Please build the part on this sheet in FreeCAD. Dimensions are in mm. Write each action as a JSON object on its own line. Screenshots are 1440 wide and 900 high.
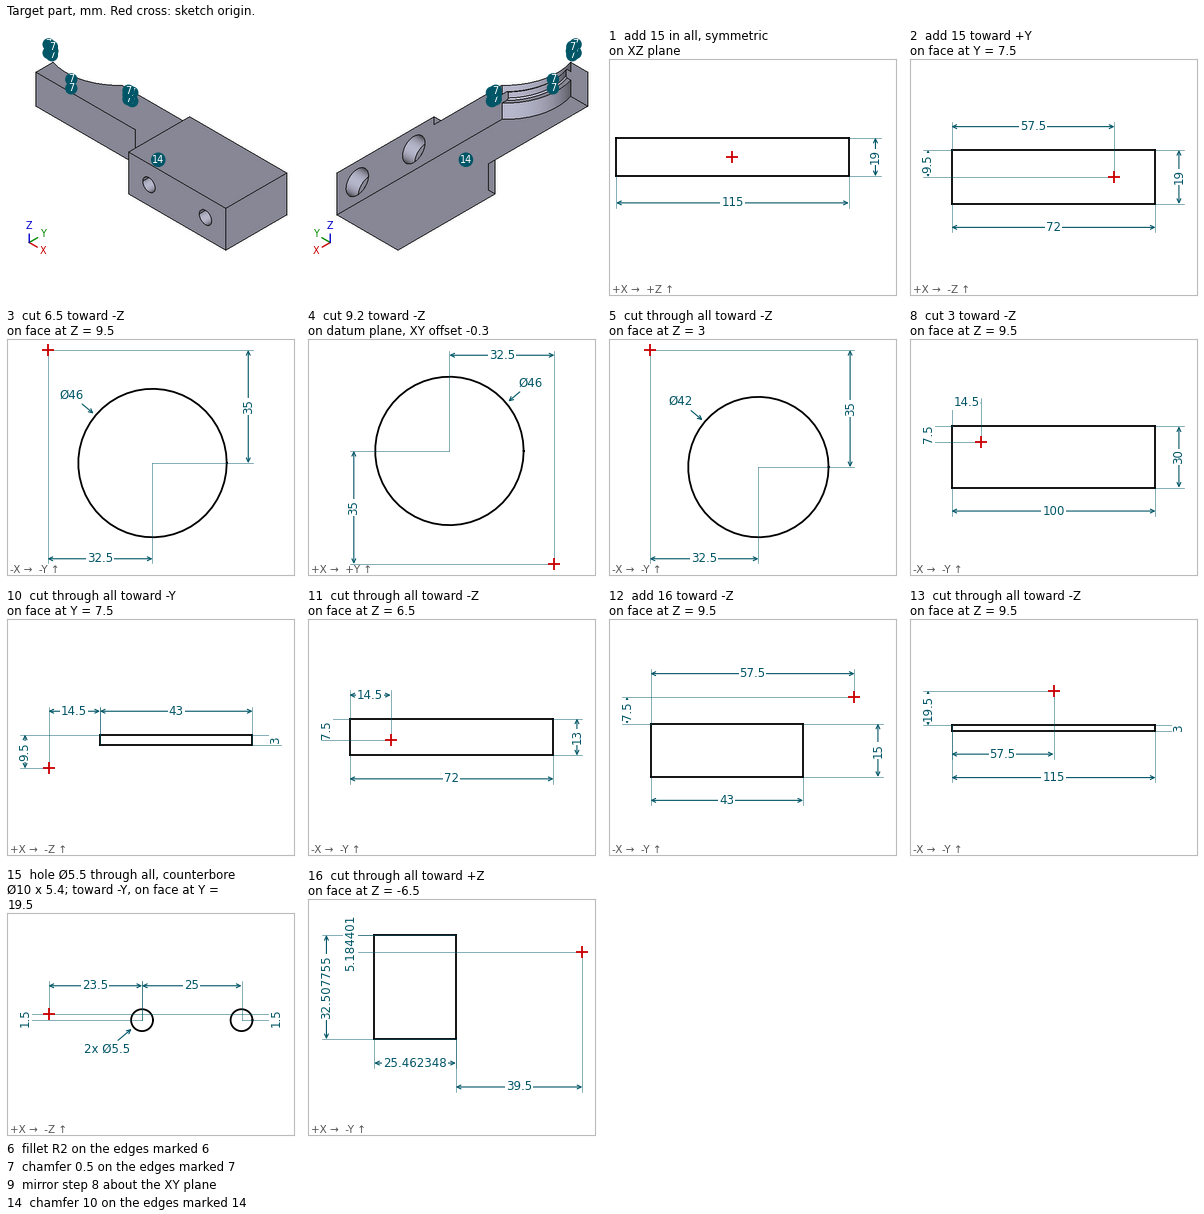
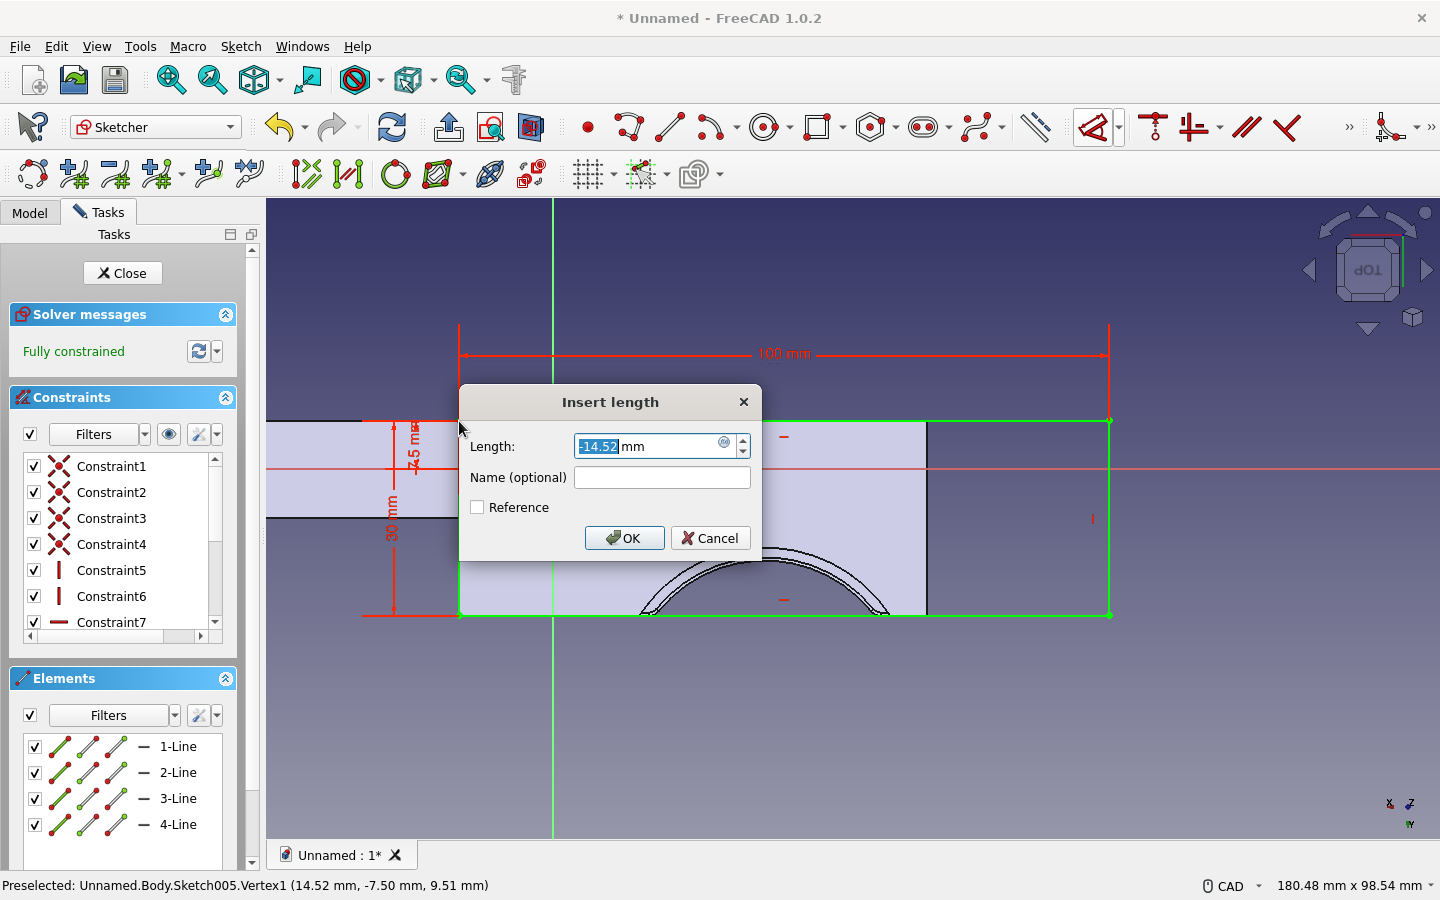
{"action": "type", "text": "-14.5"}
{"action": "key", "text": "Return"}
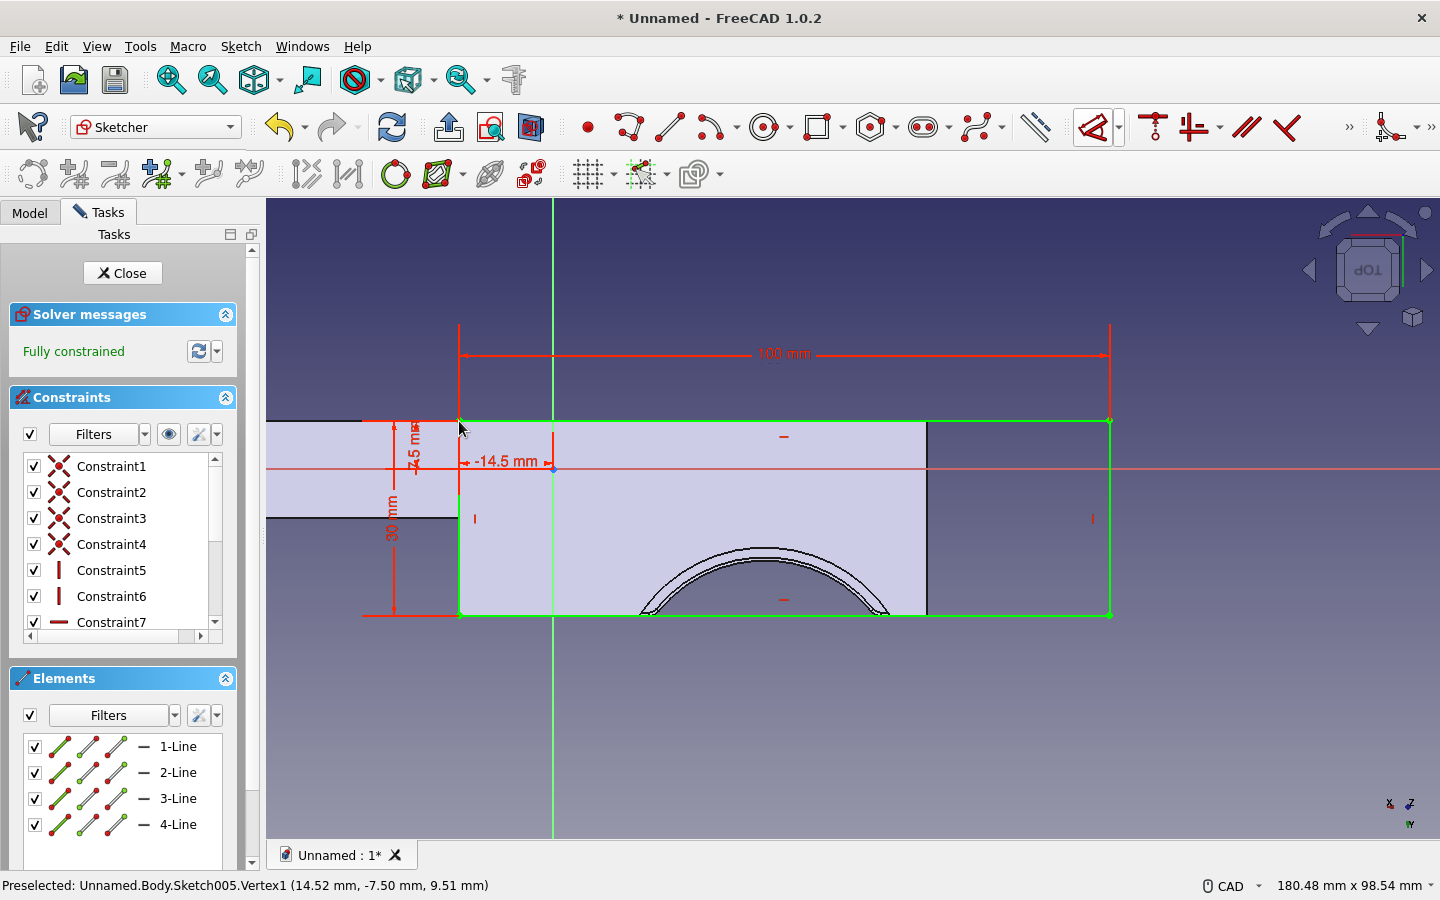
{"action": "left_click", "coordinate": [123, 273]}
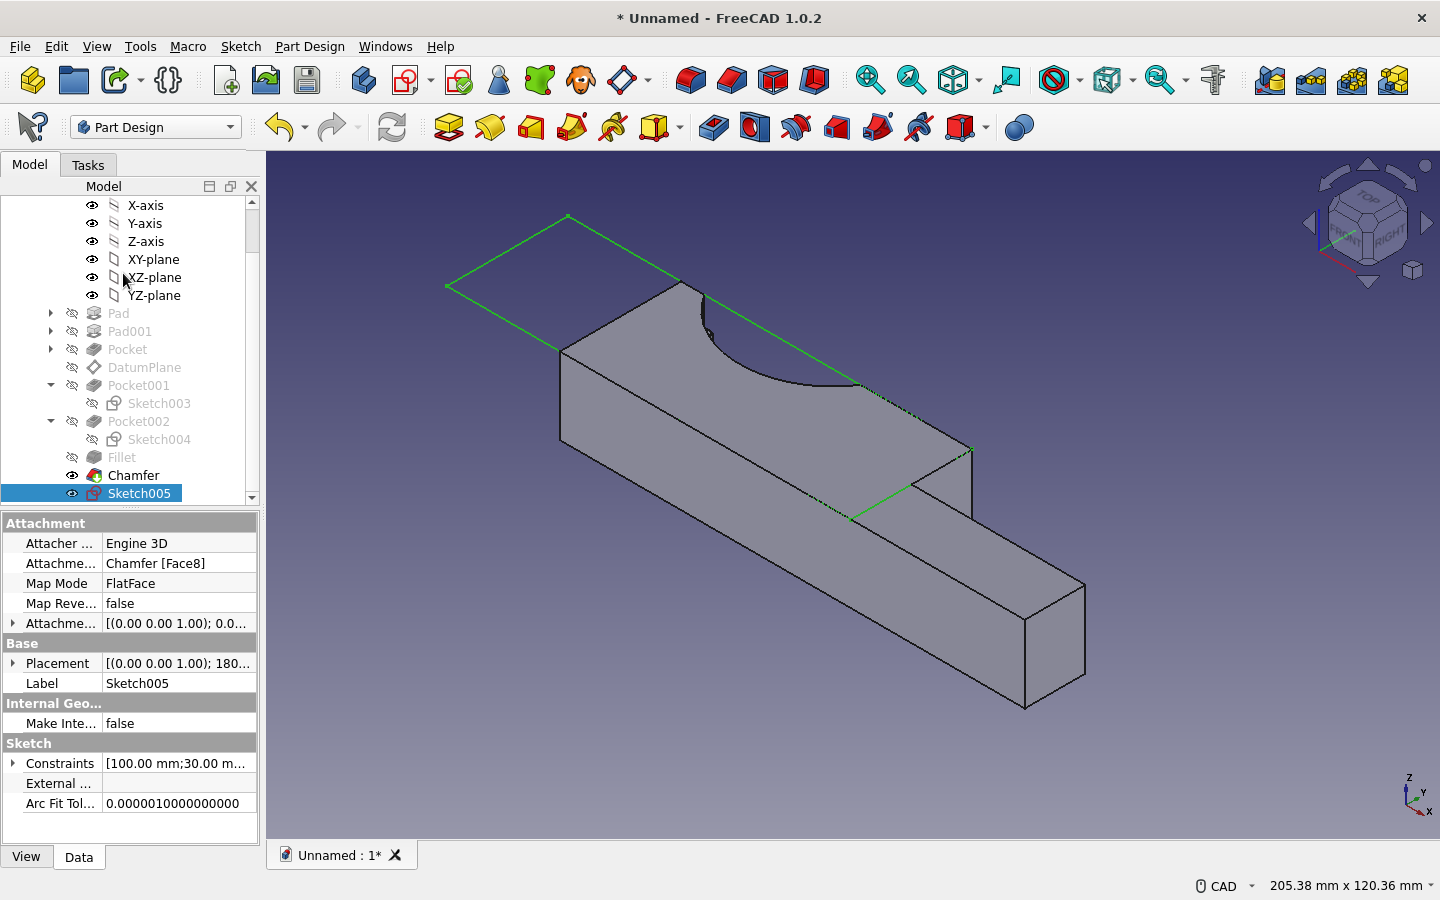
{"action": "left_click", "coordinate": [714, 128]}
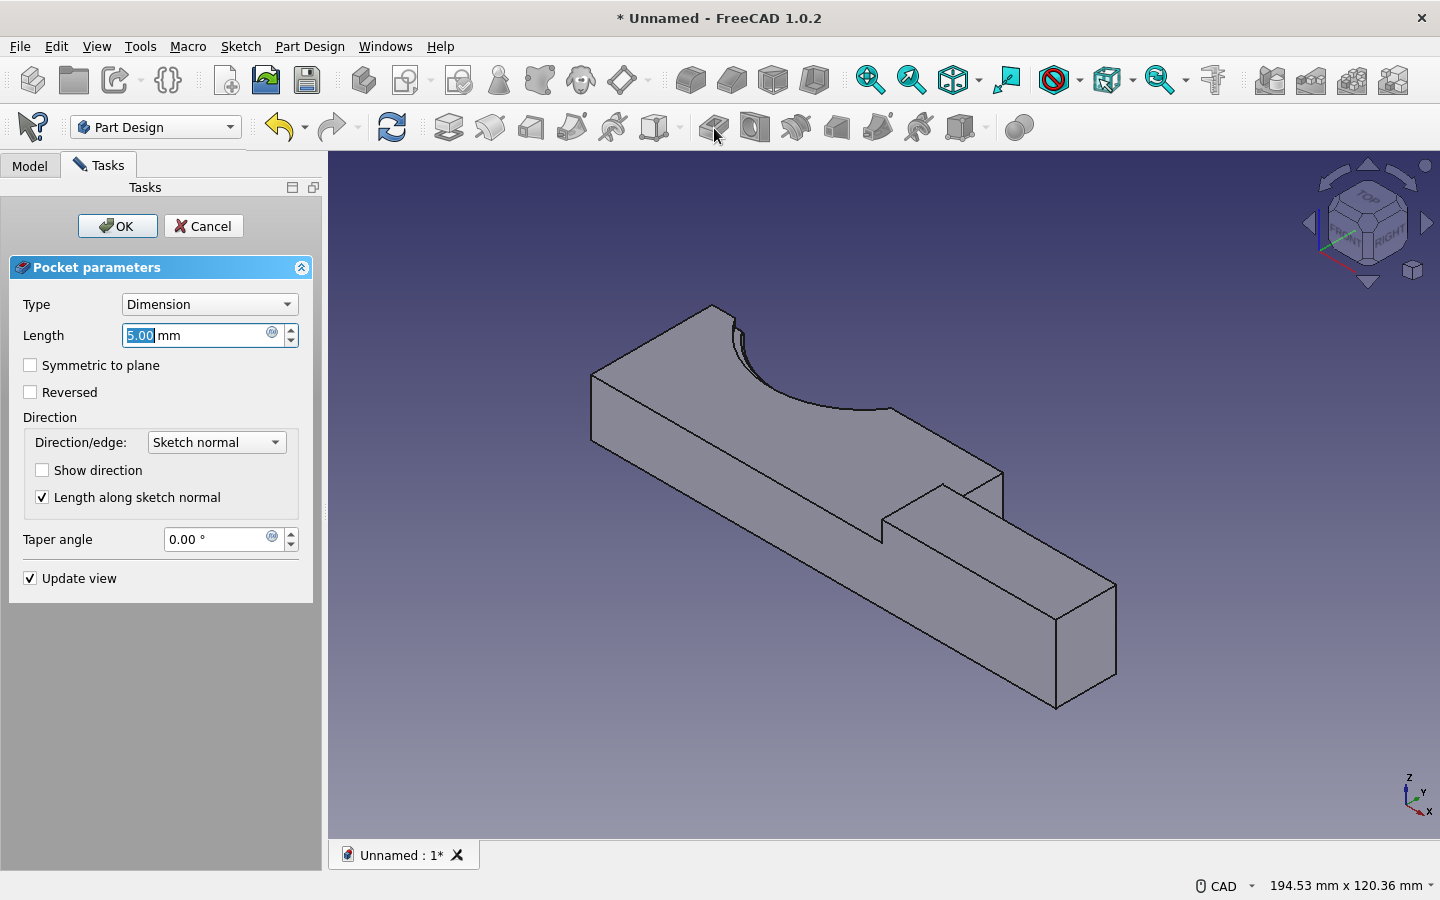
{"action": "type", "text": "3"}
{"action": "key", "text": "Tab"}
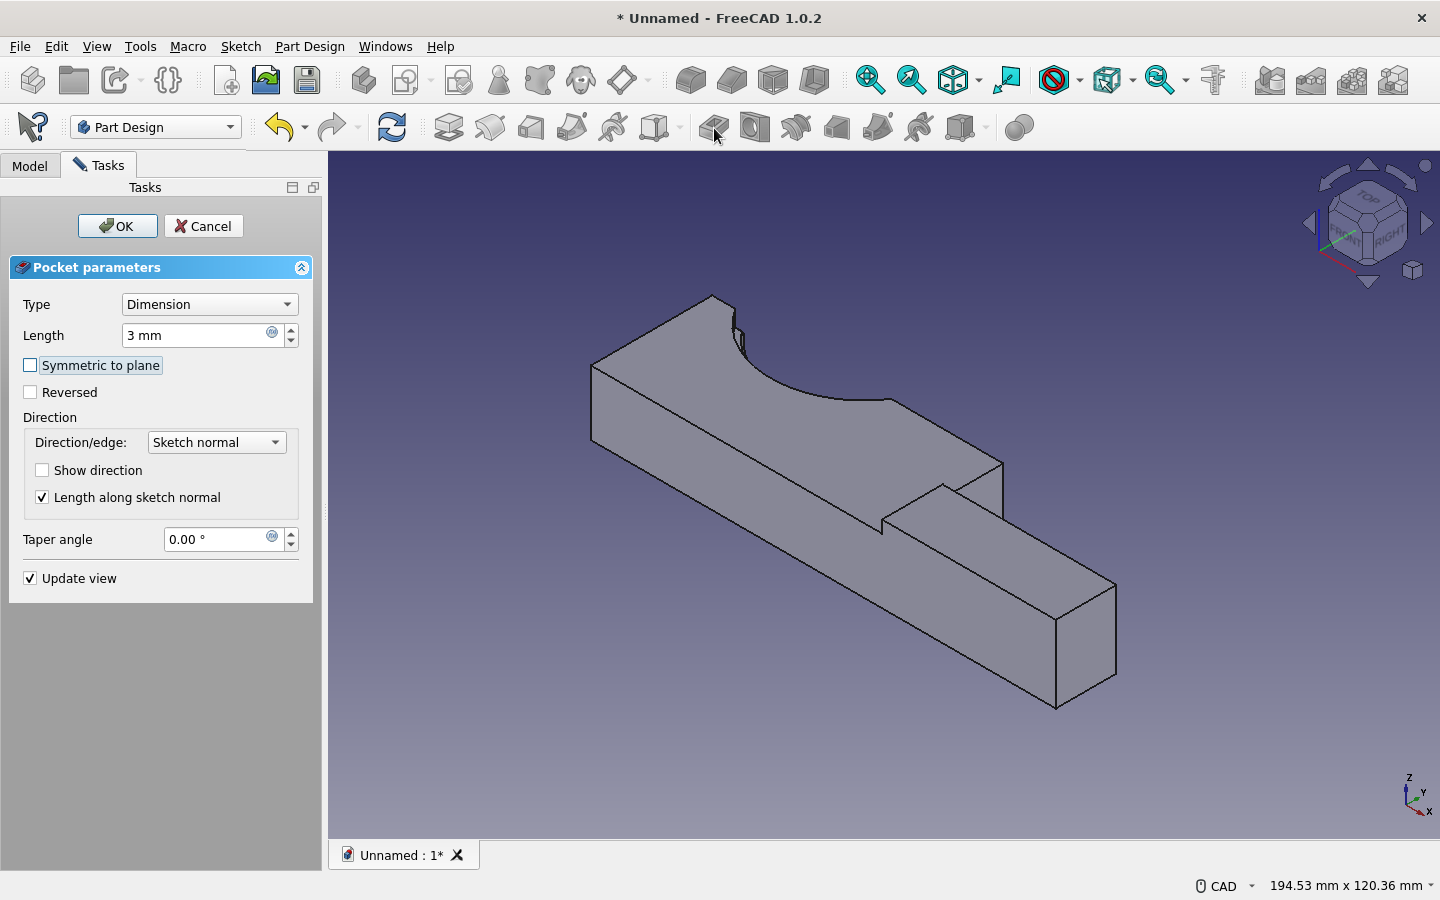
{"action": "left_click", "coordinate": [118, 226]}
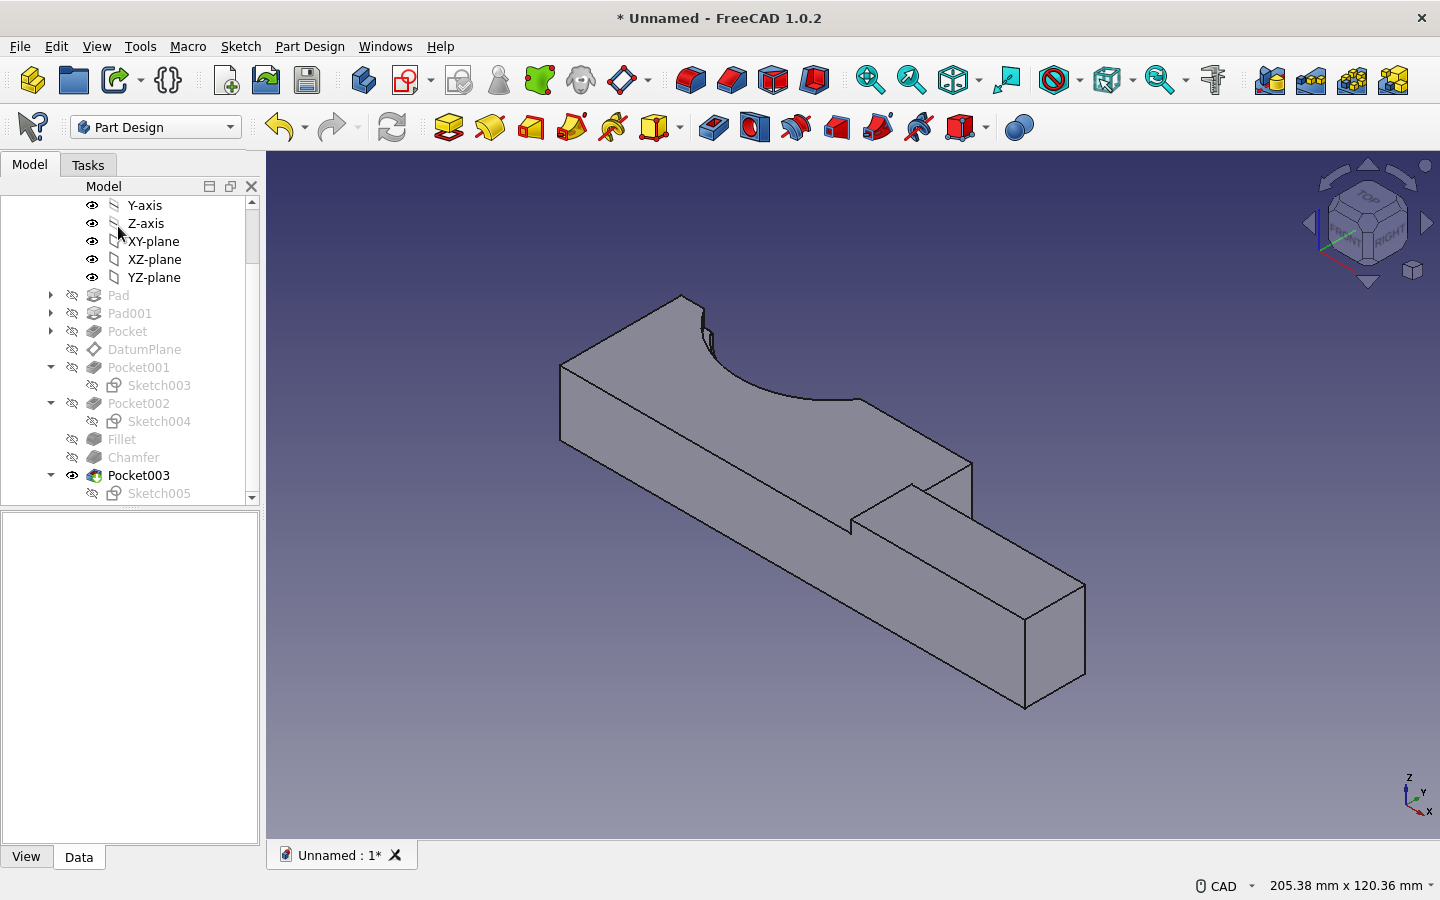
{"action": "left_click", "coordinate": [117, 475]}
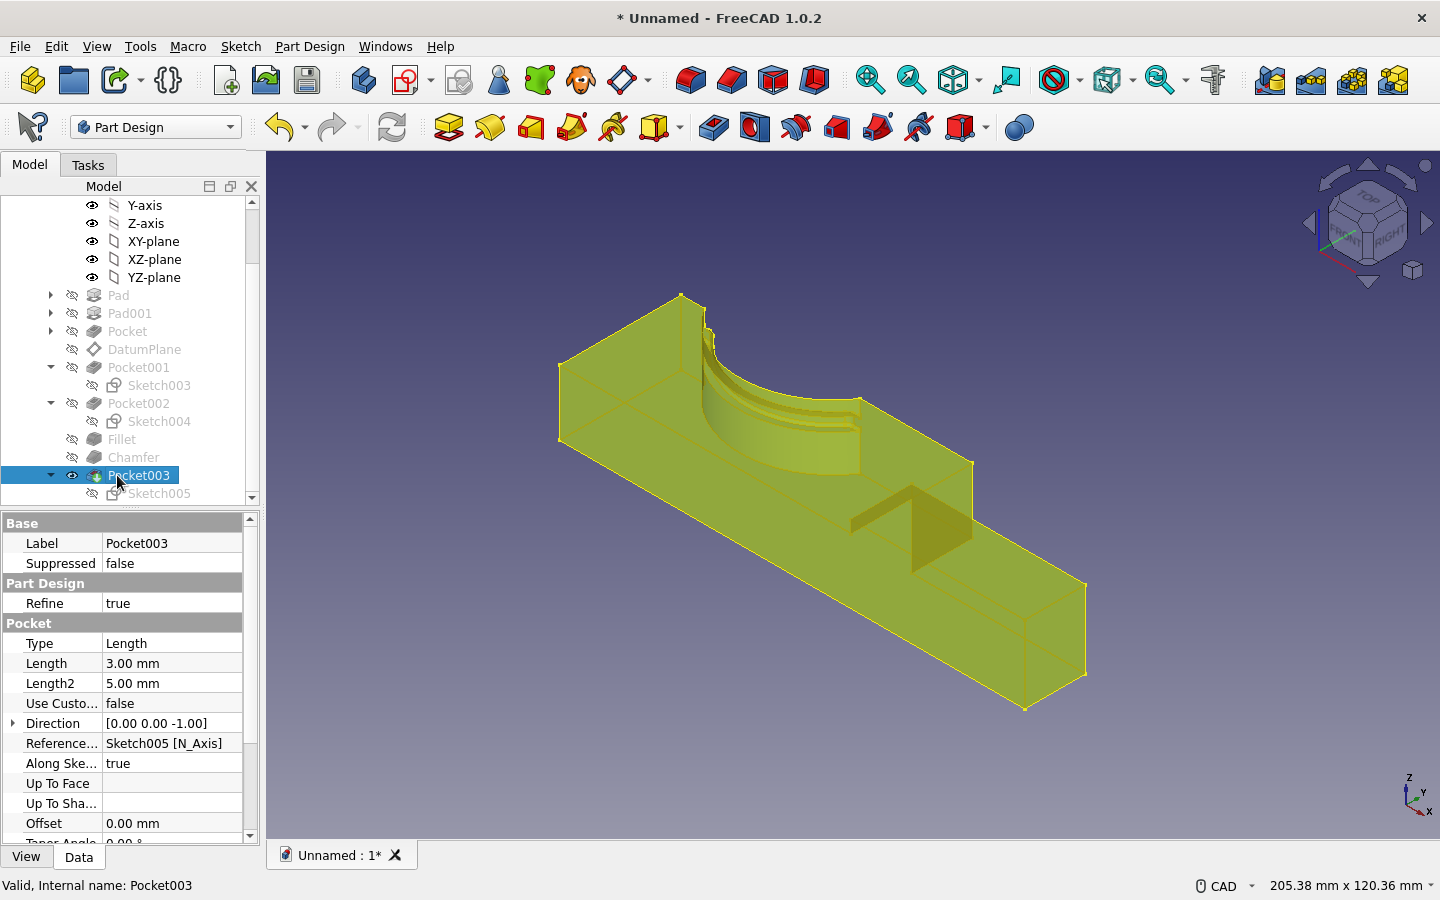
{"action": "left_click", "coordinate": [1270, 80]}